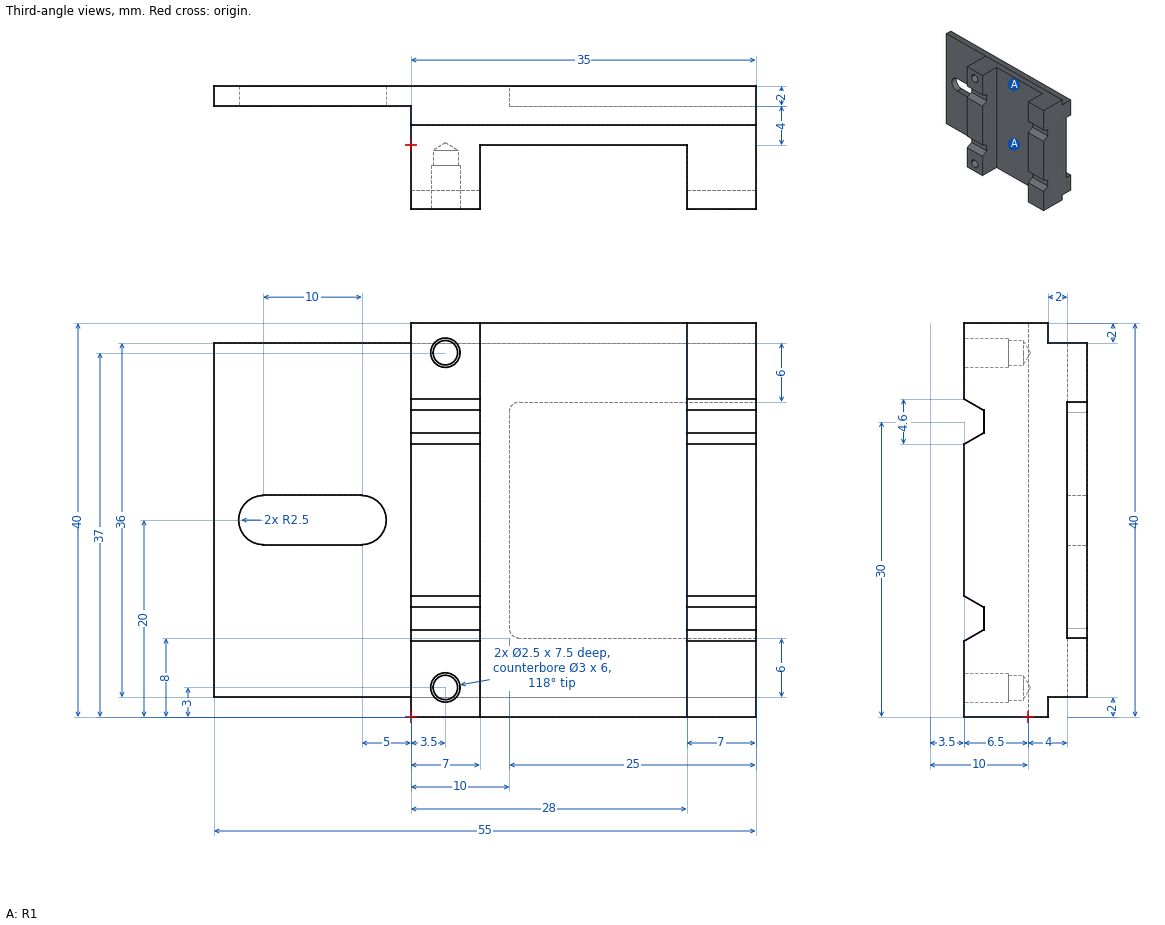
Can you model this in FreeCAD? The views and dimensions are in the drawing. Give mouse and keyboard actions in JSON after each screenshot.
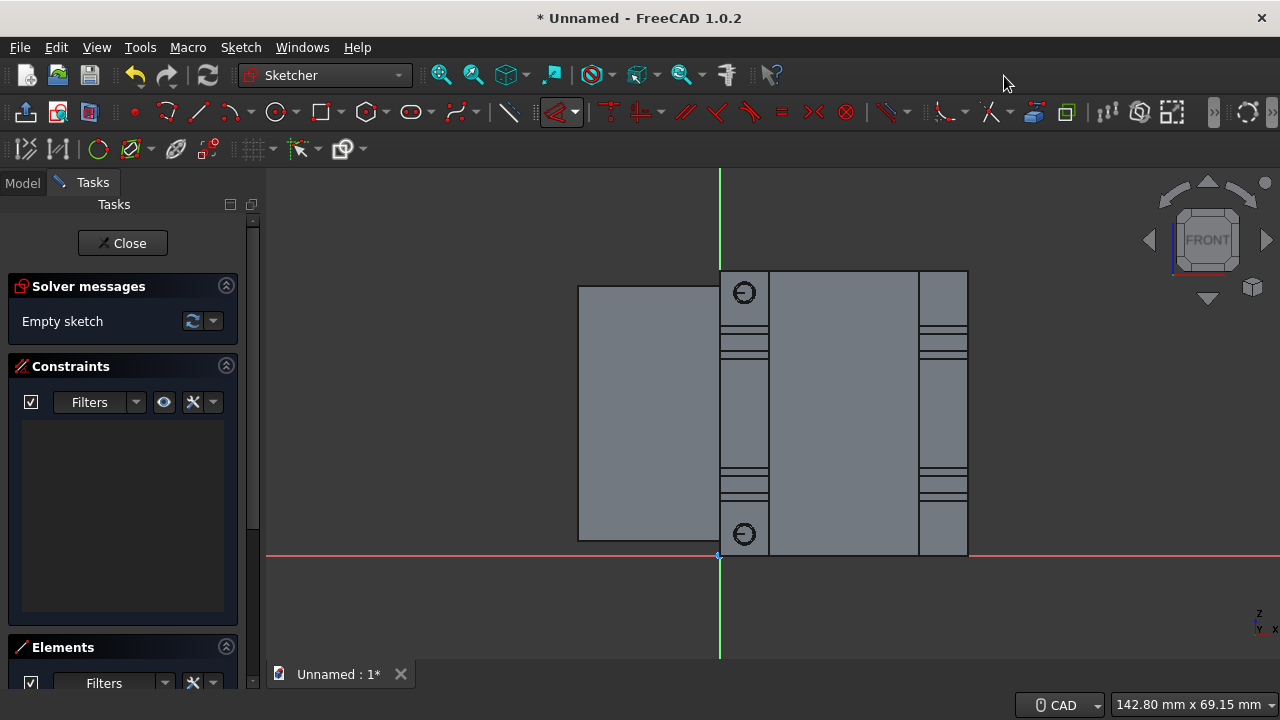
{"action": "scroll", "coordinate": [601, 551], "scroll_direction": "up", "scroll_amount": 3}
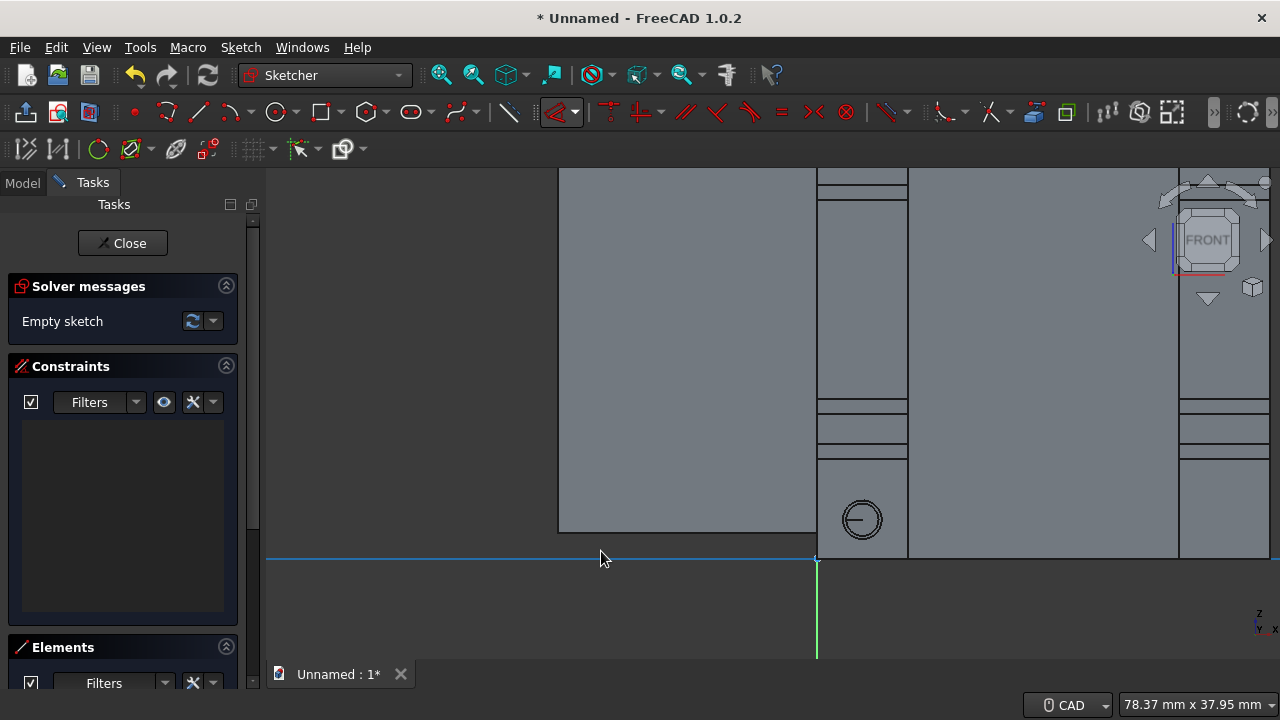
{"action": "left_click", "coordinate": [412, 112]}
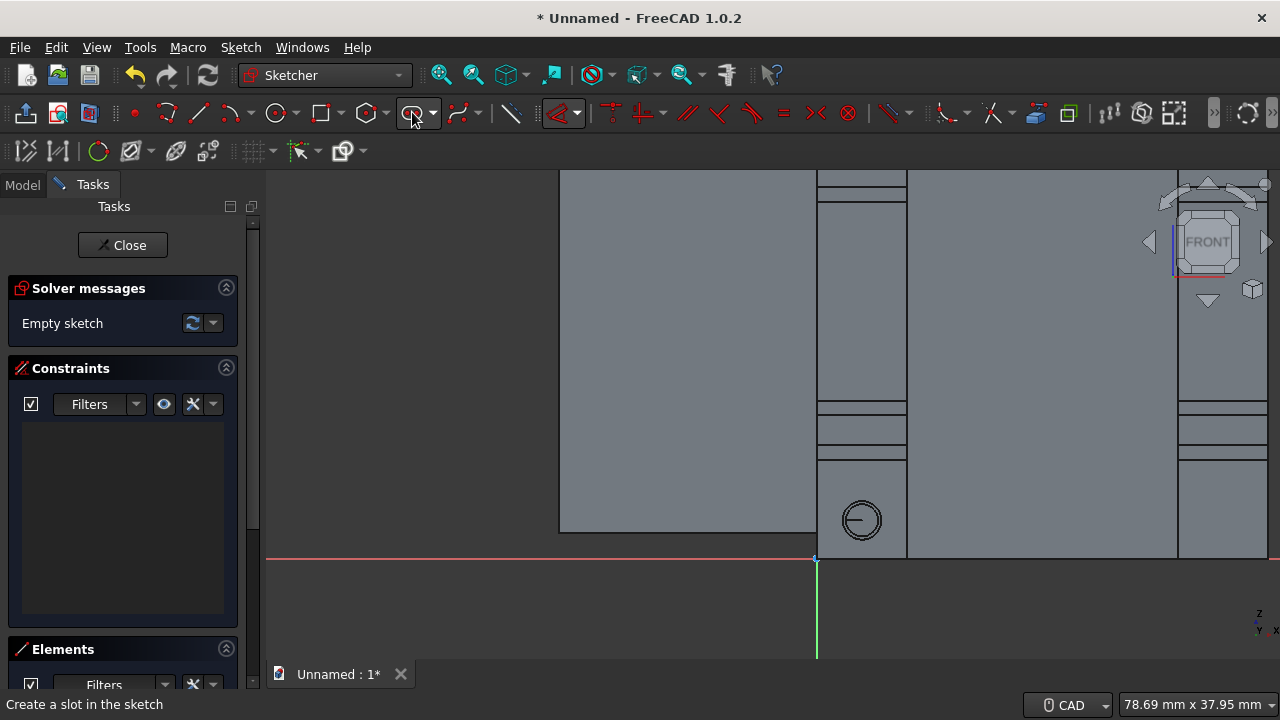
{"action": "left_click", "coordinate": [624, 301]}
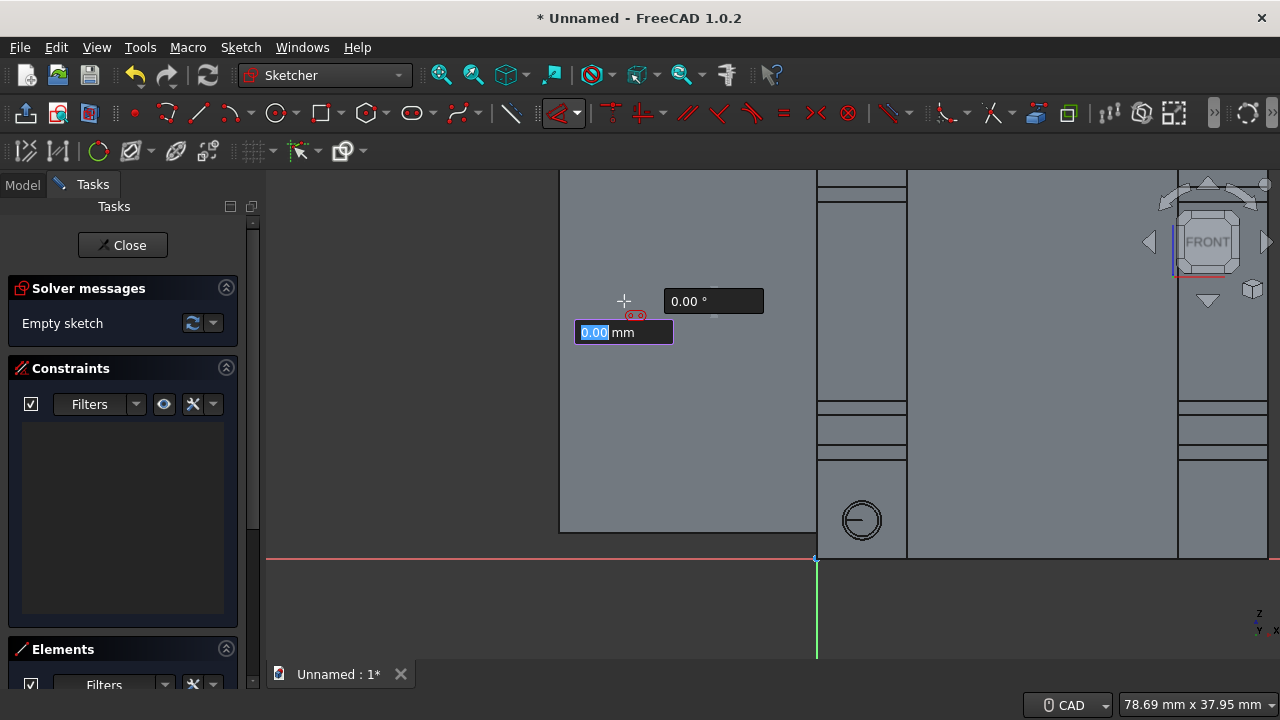
{"action": "left_click", "coordinate": [752, 301]}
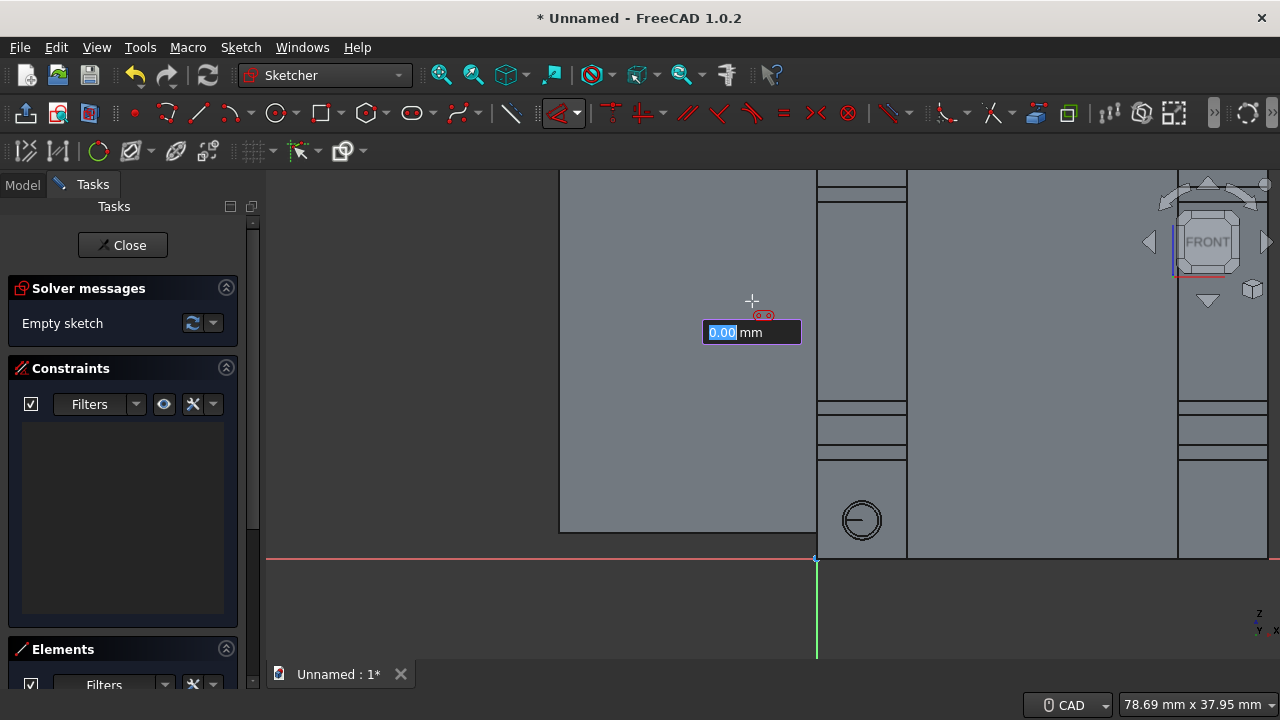
{"action": "left_click", "coordinate": [688, 269]}
{"action": "key", "text": "Escape"}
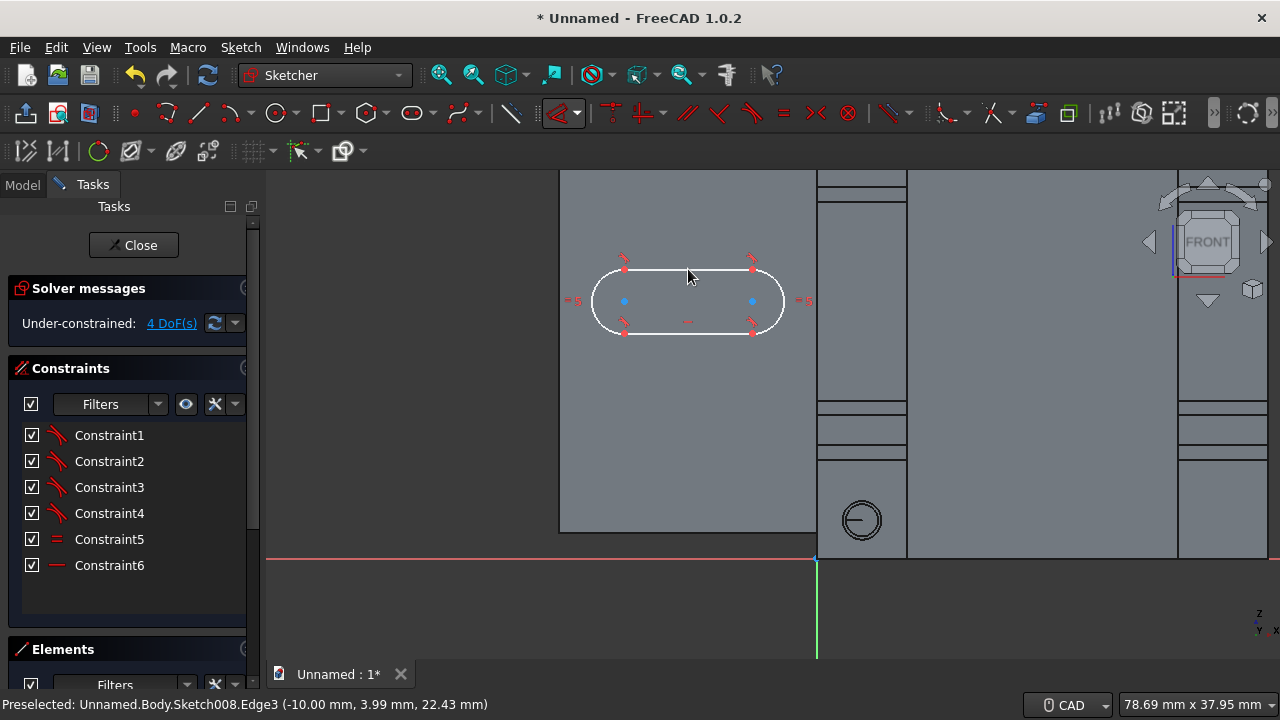
{"action": "scroll", "coordinate": [598, 283], "scroll_direction": "up", "scroll_amount": 2}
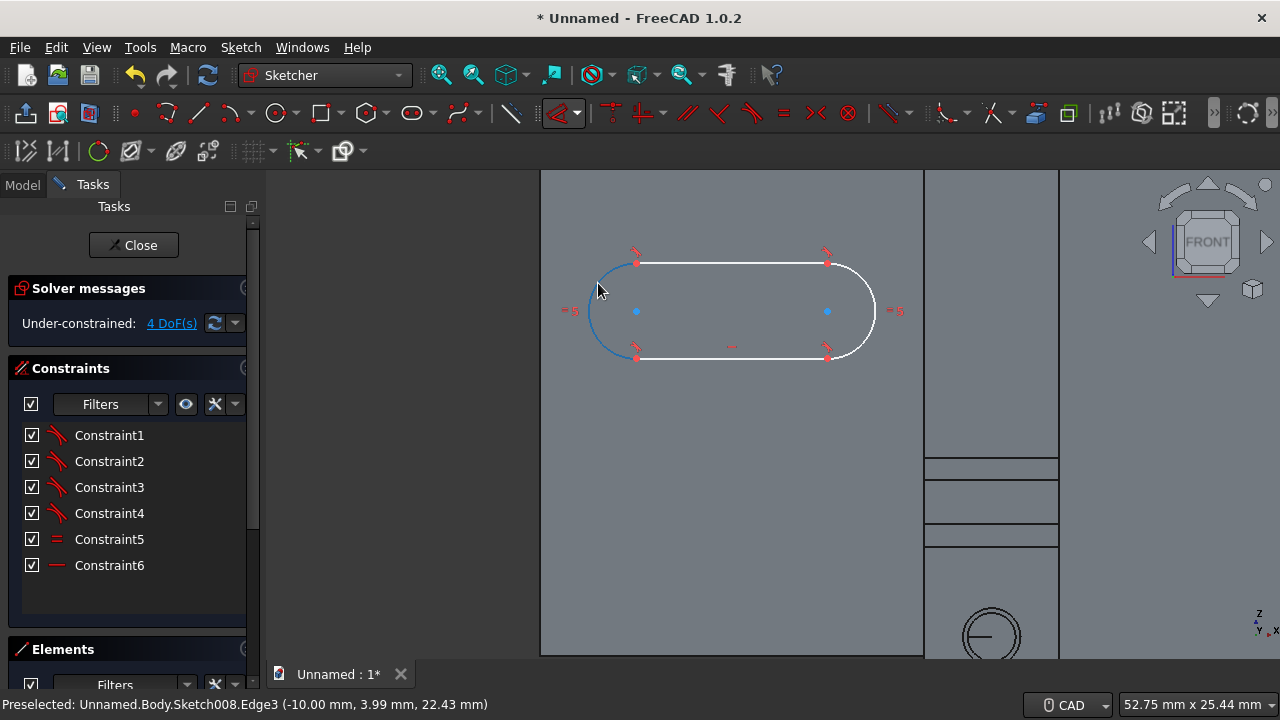
{"action": "left_click", "coordinate": [598, 283]}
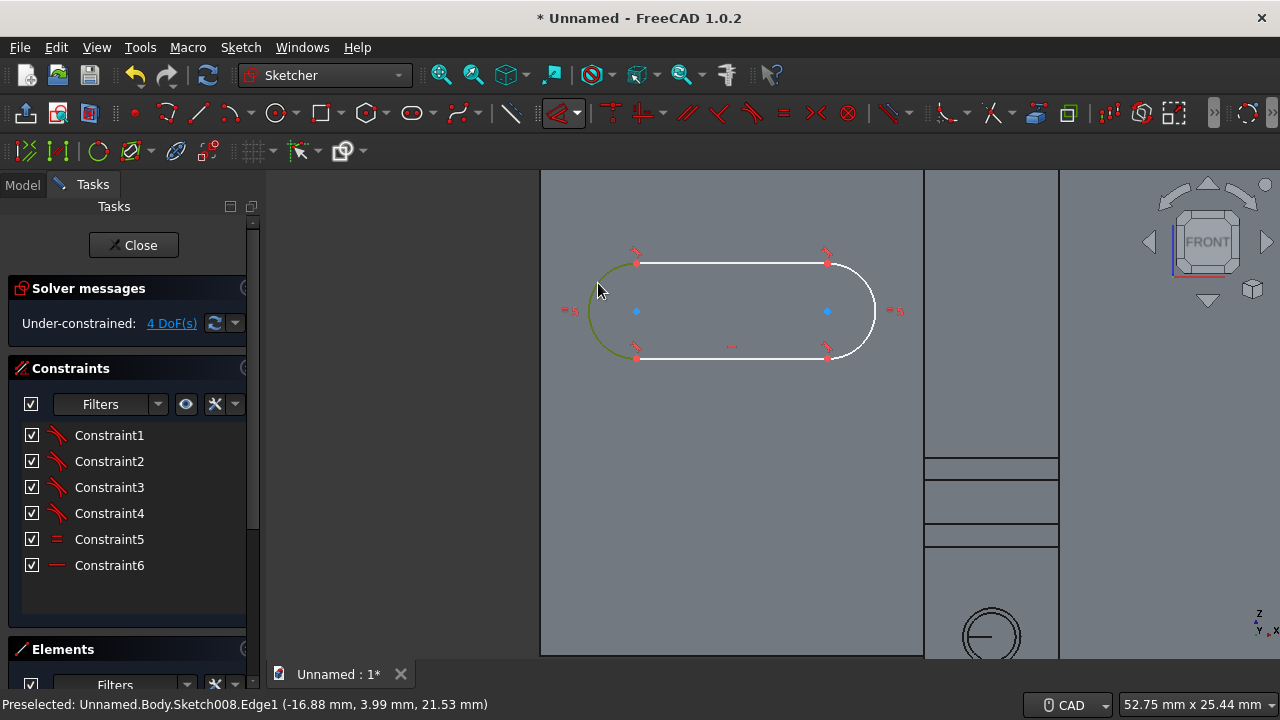
{"action": "key", "text": "k r"}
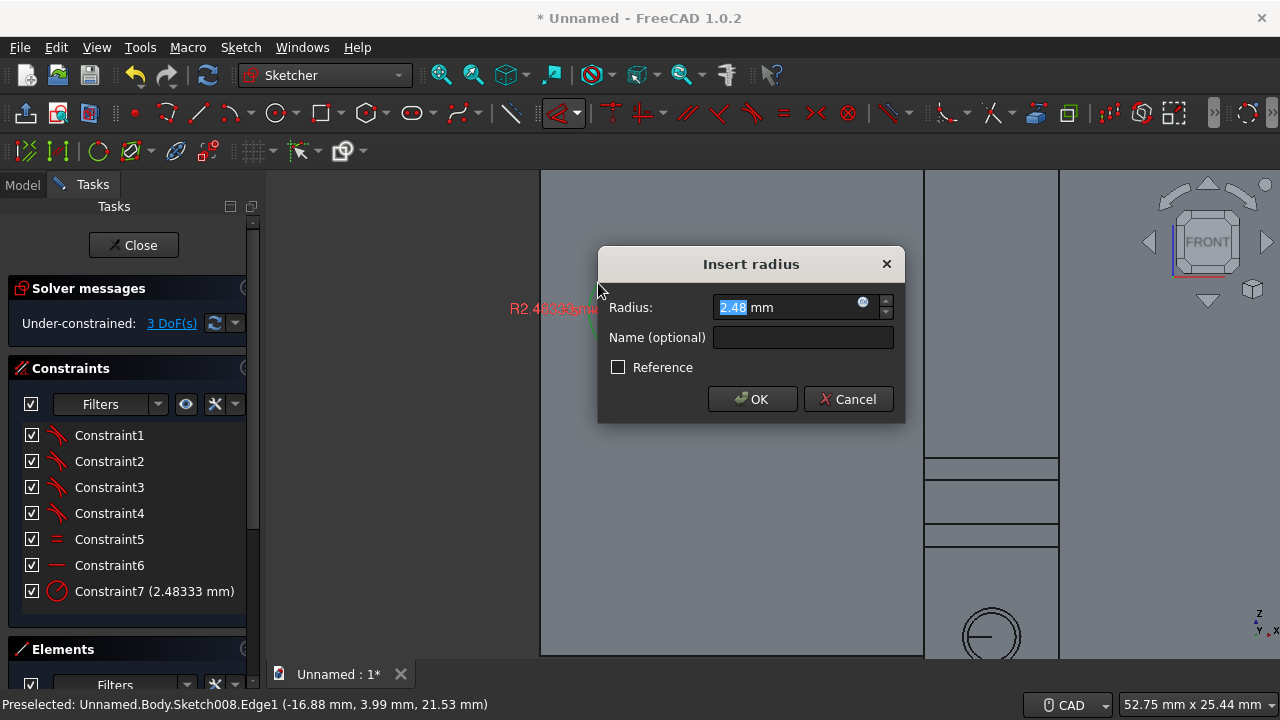
{"action": "type", "text": "2.5"}
{"action": "key", "text": "Return"}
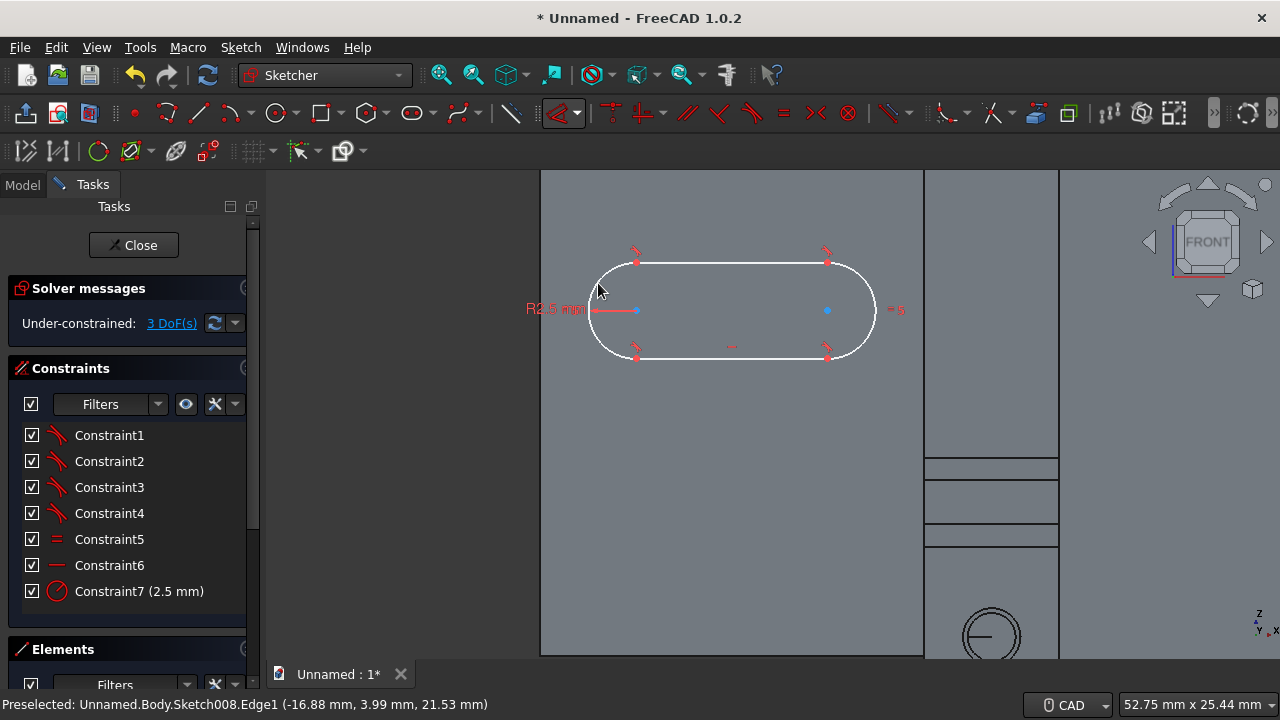
{"action": "left_click", "coordinate": [694, 263]}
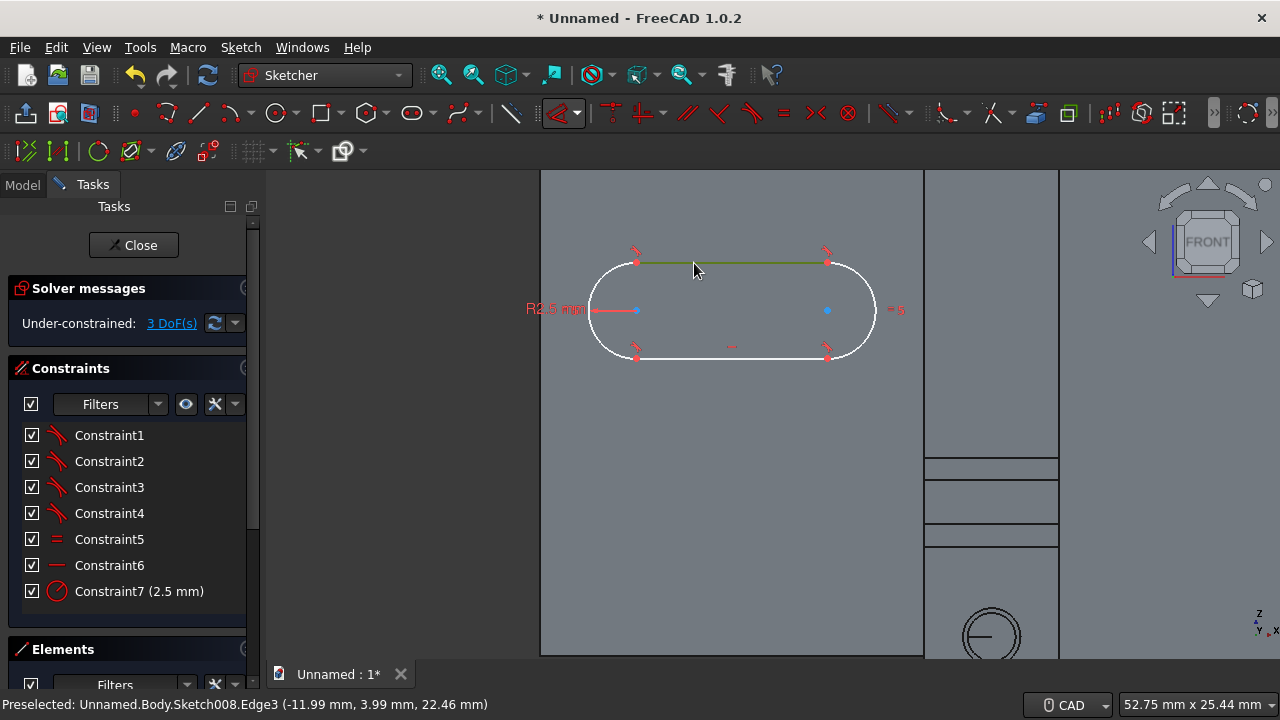
{"action": "left_click", "coordinate": [580, 114]}